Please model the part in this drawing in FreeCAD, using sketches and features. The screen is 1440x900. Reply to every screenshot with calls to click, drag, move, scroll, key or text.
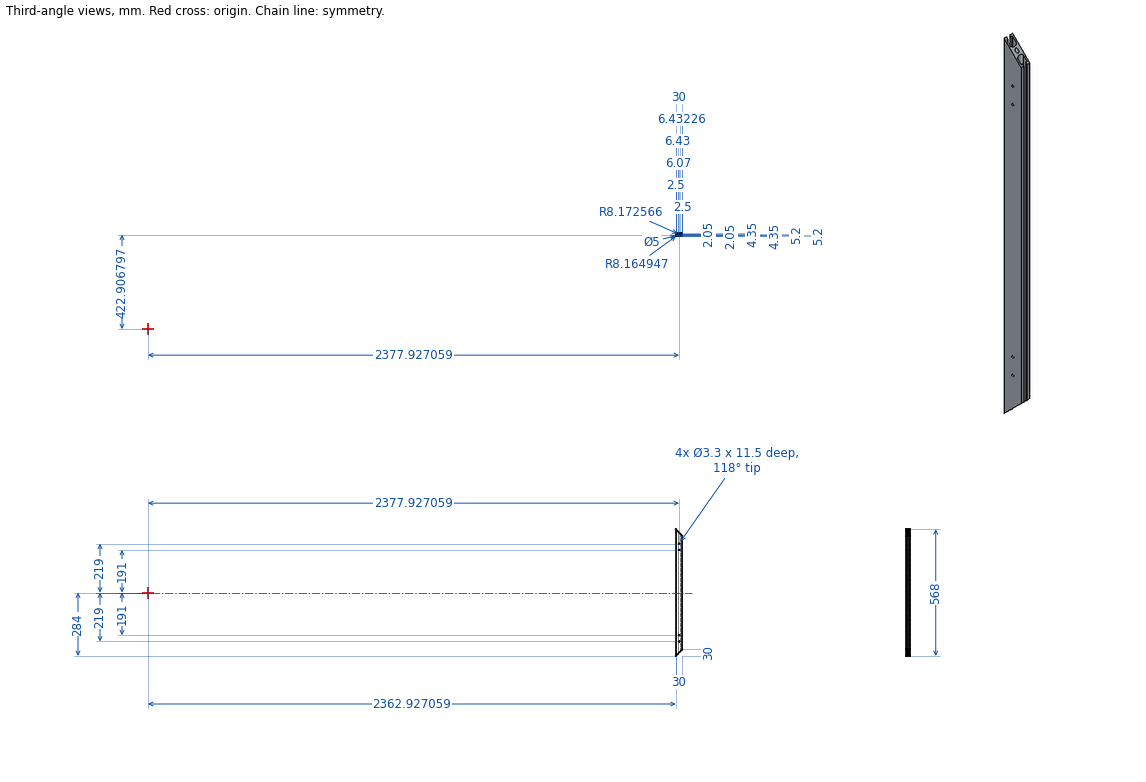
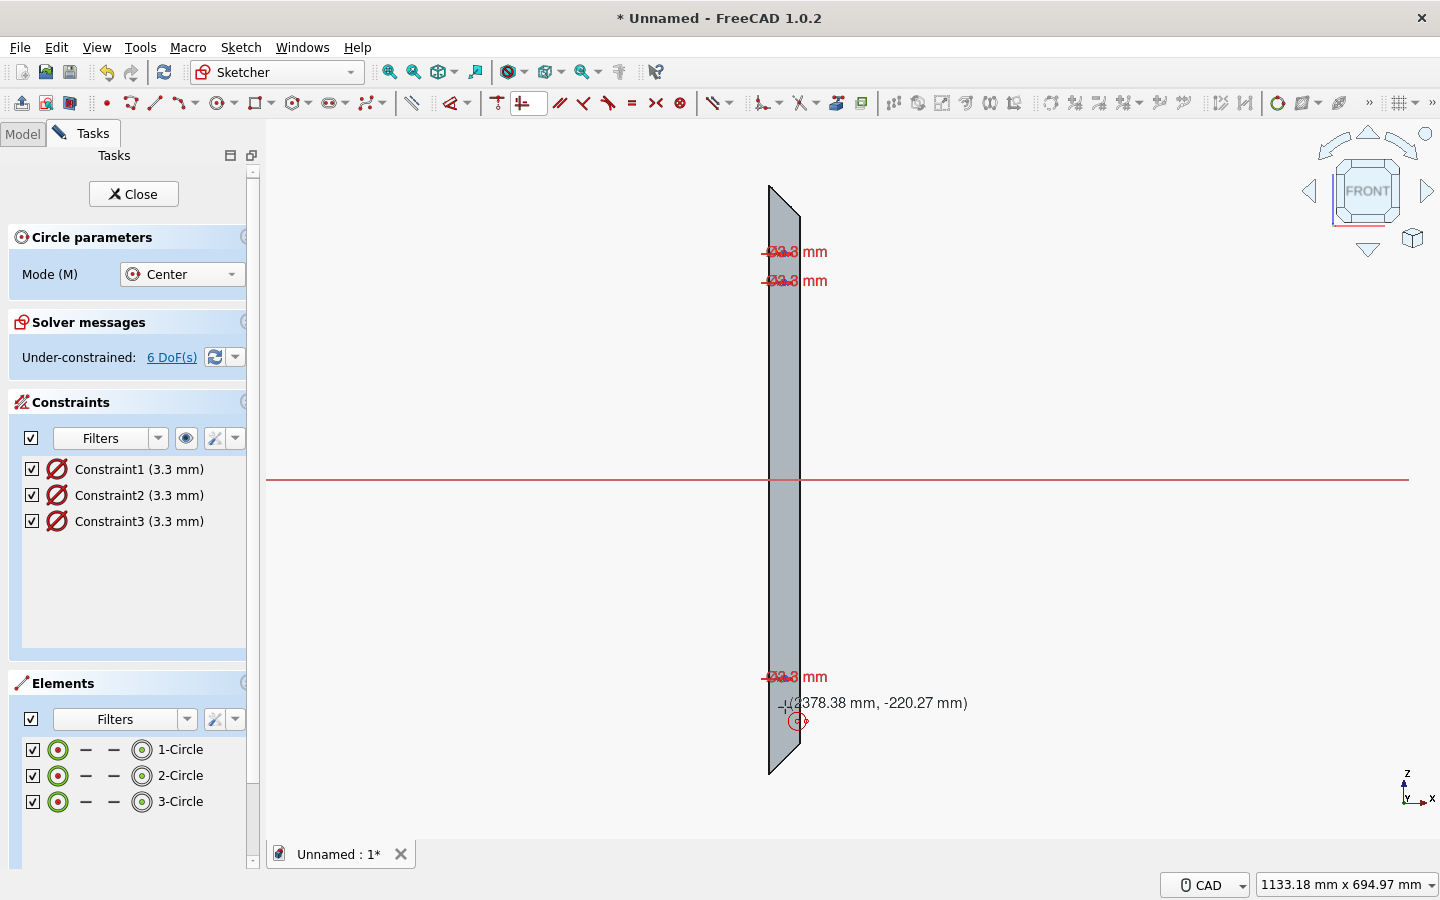
click(785, 707)
move(786, 705)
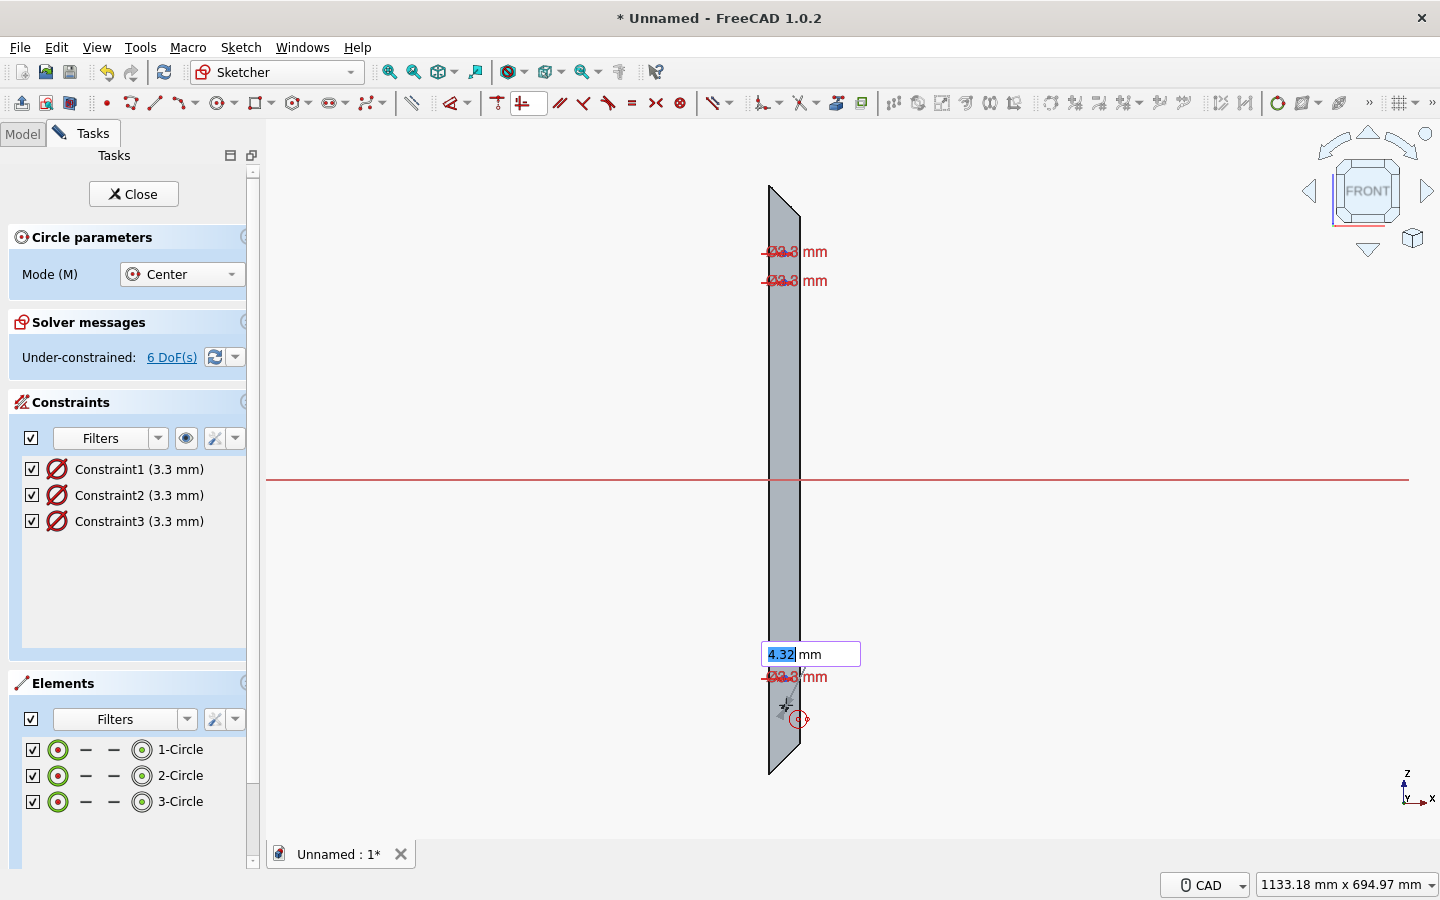
text(3.3)
key(Return)
key(Escape)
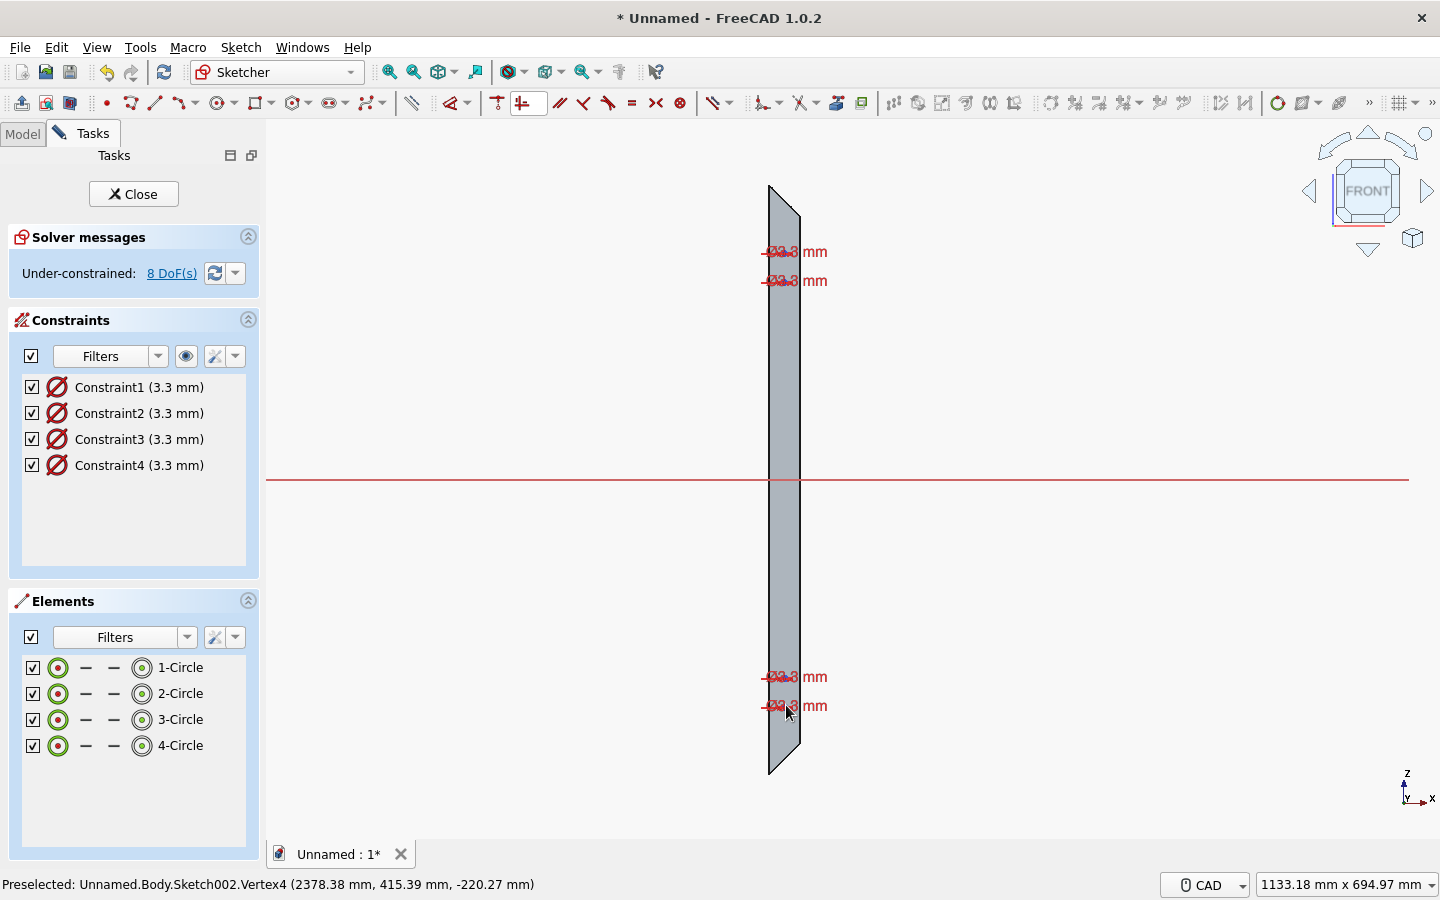
click(785, 254)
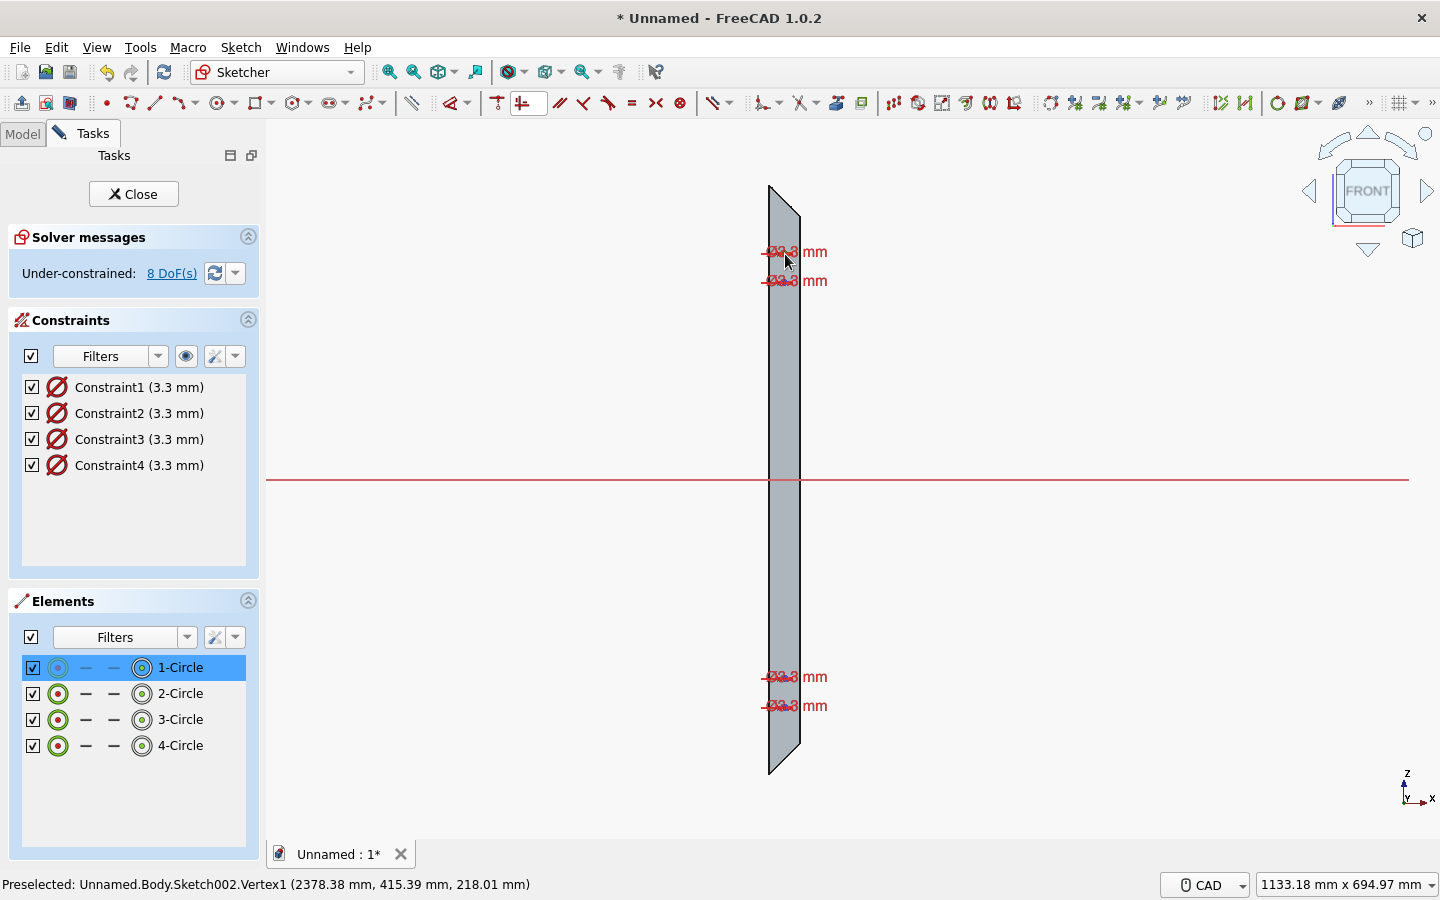
click(785, 283)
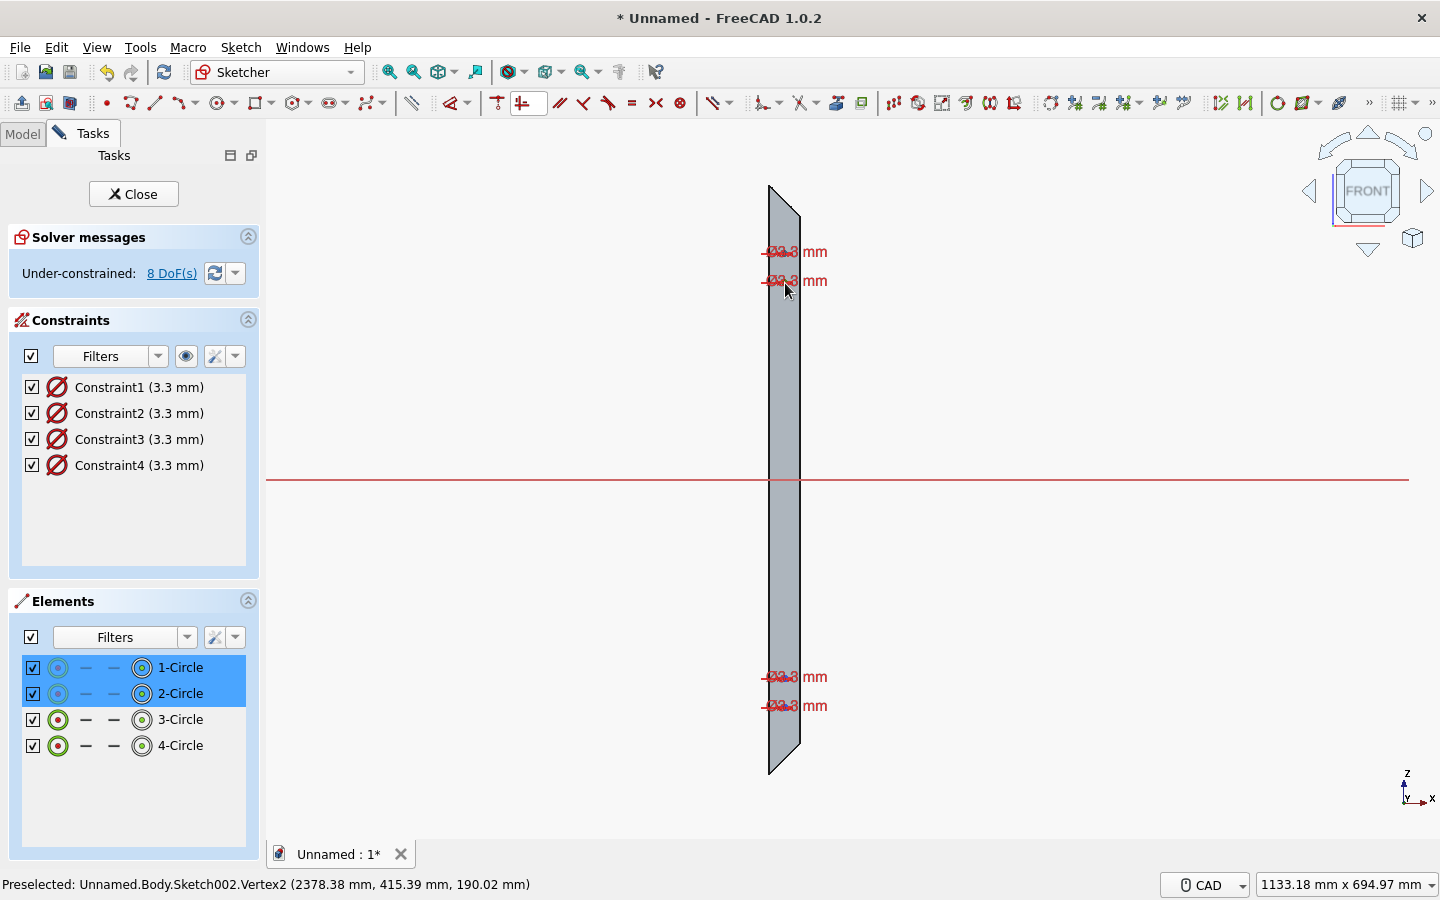
click(542, 104)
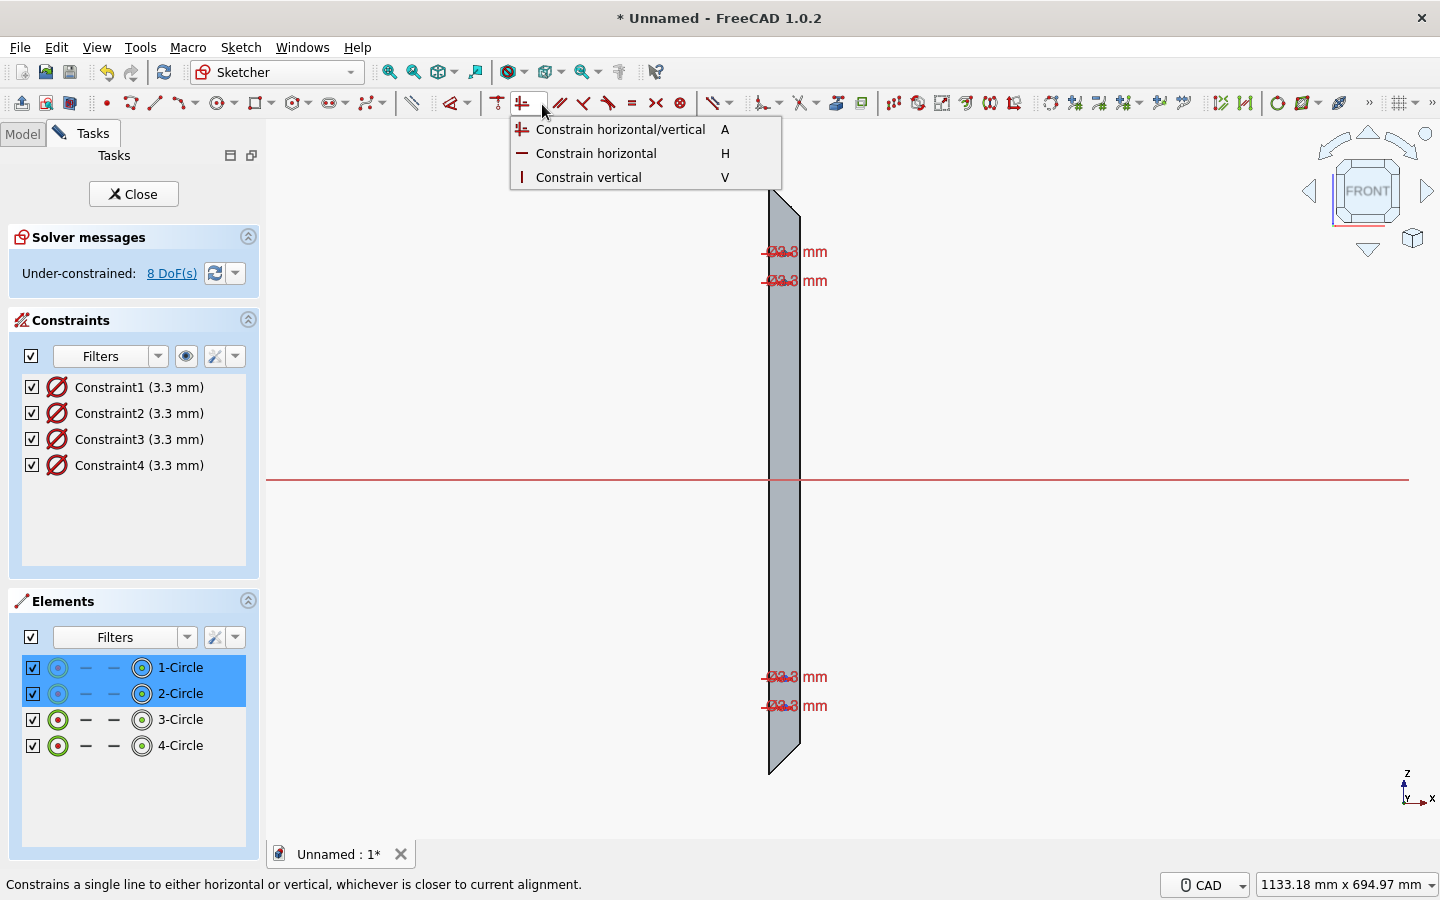
click(646, 177)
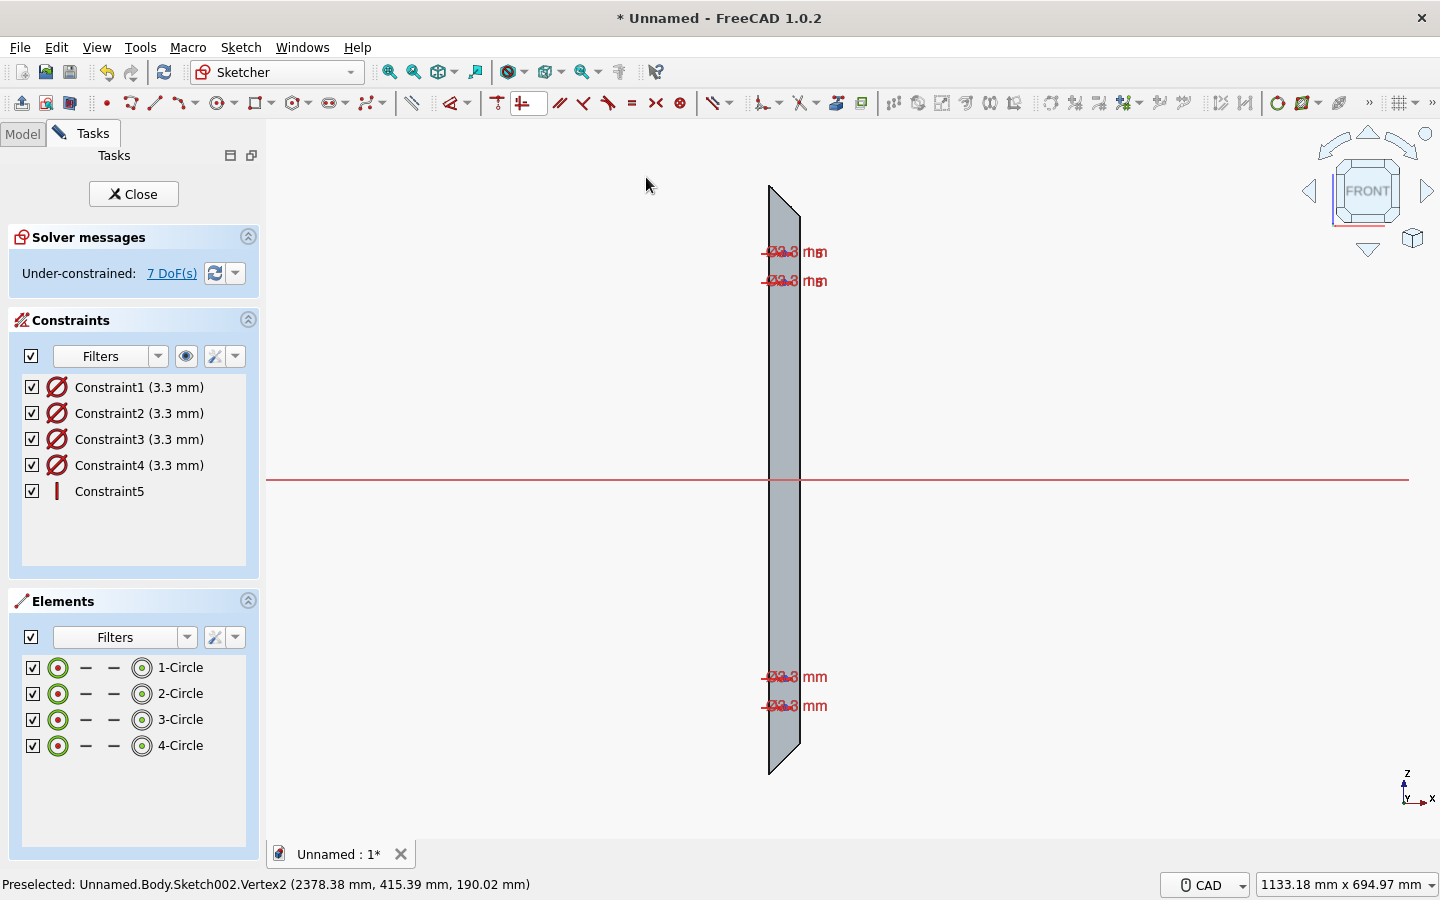
click(785, 283)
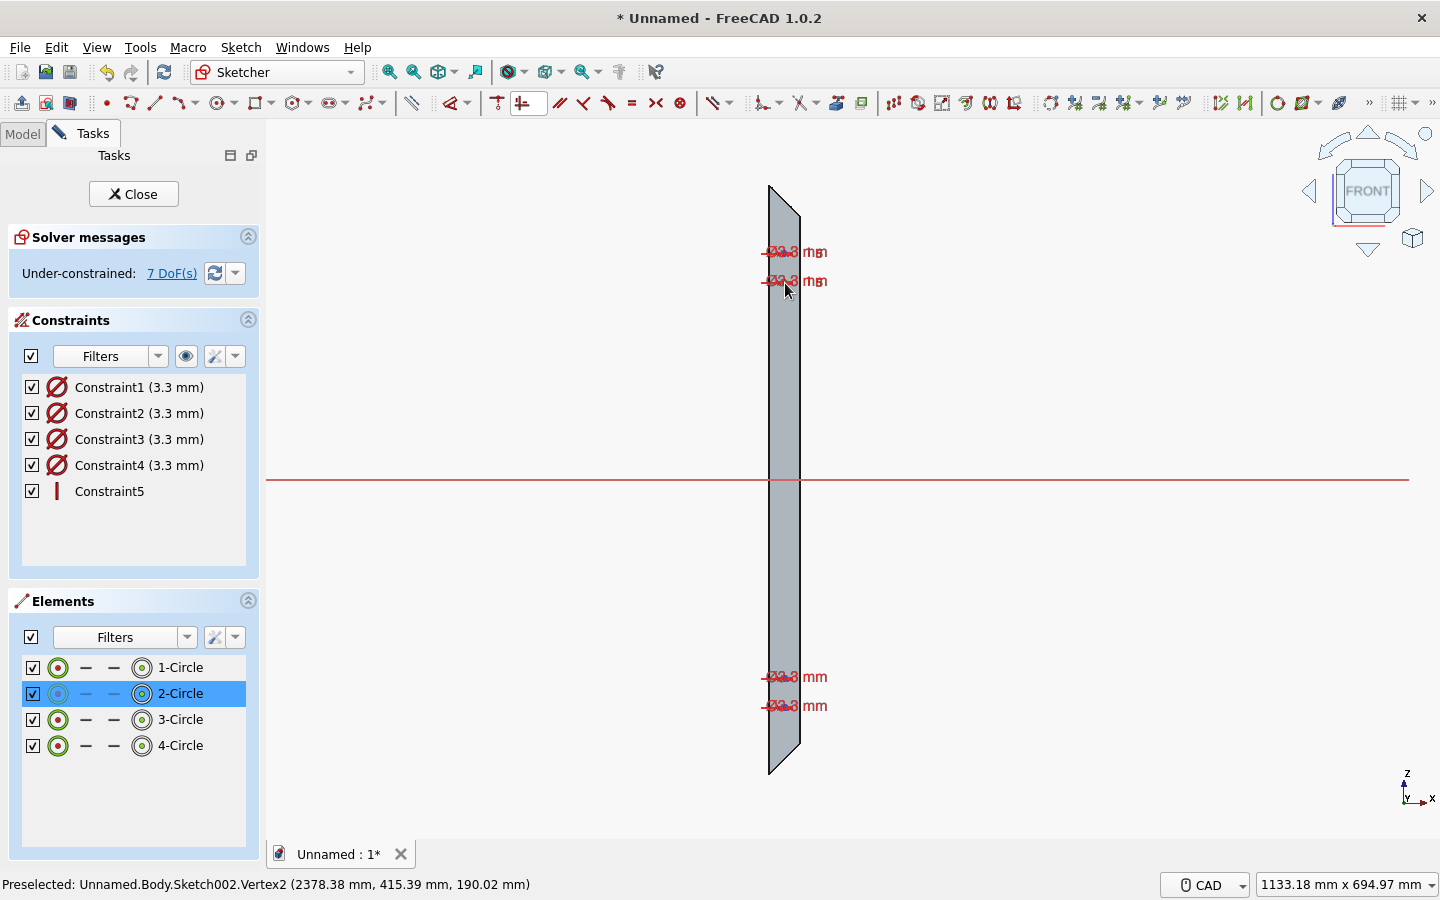
click(785, 679)